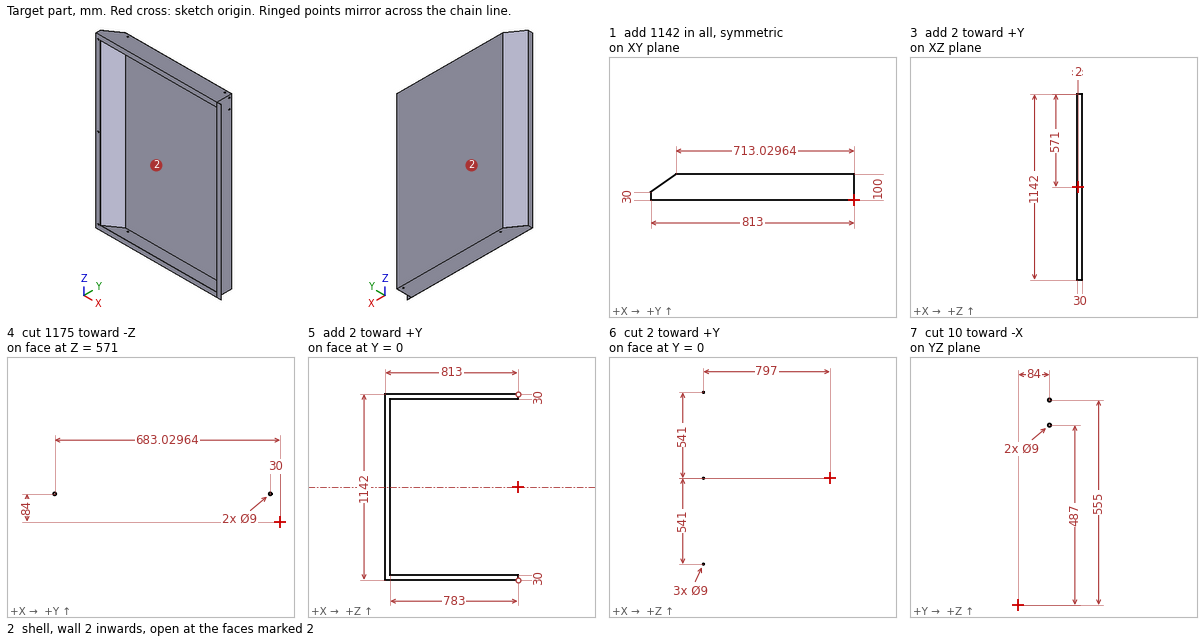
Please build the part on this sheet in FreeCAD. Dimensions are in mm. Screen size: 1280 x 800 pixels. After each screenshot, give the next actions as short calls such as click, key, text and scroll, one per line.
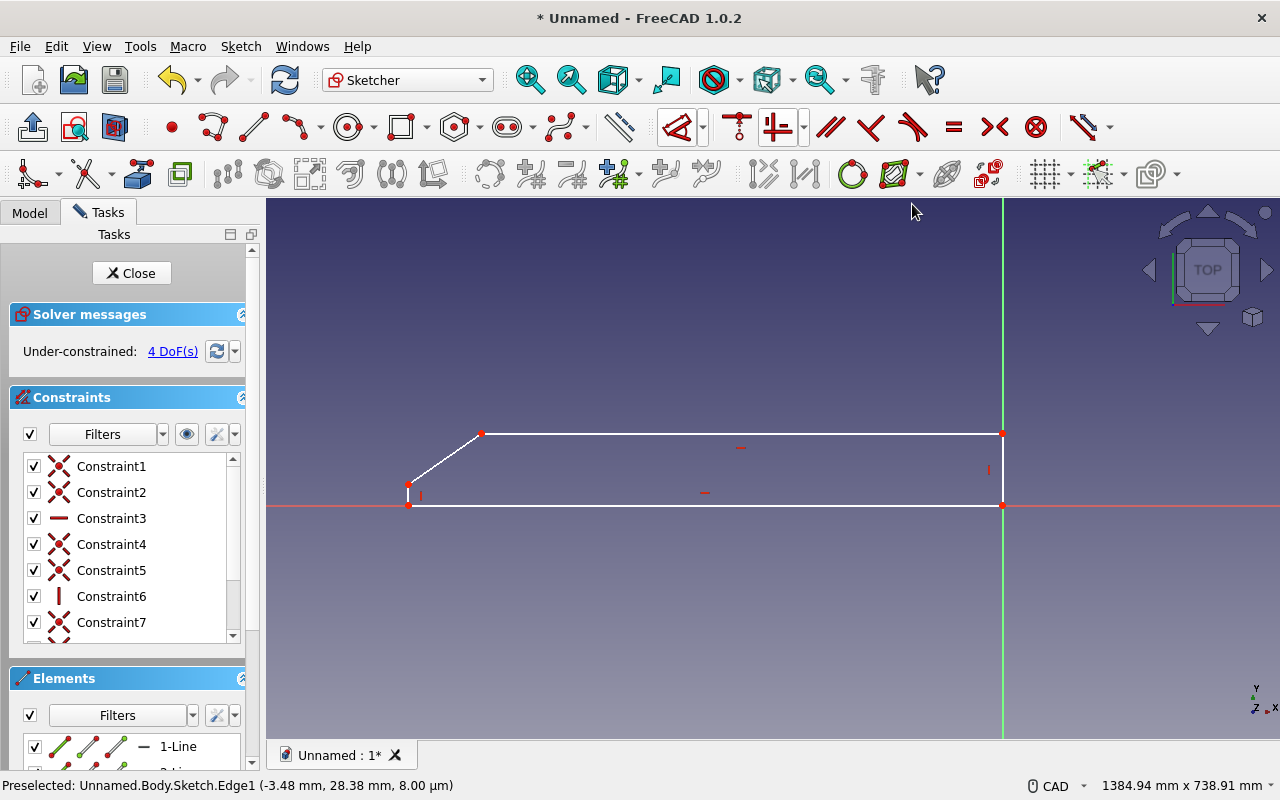
scroll(408, 495, up, 3)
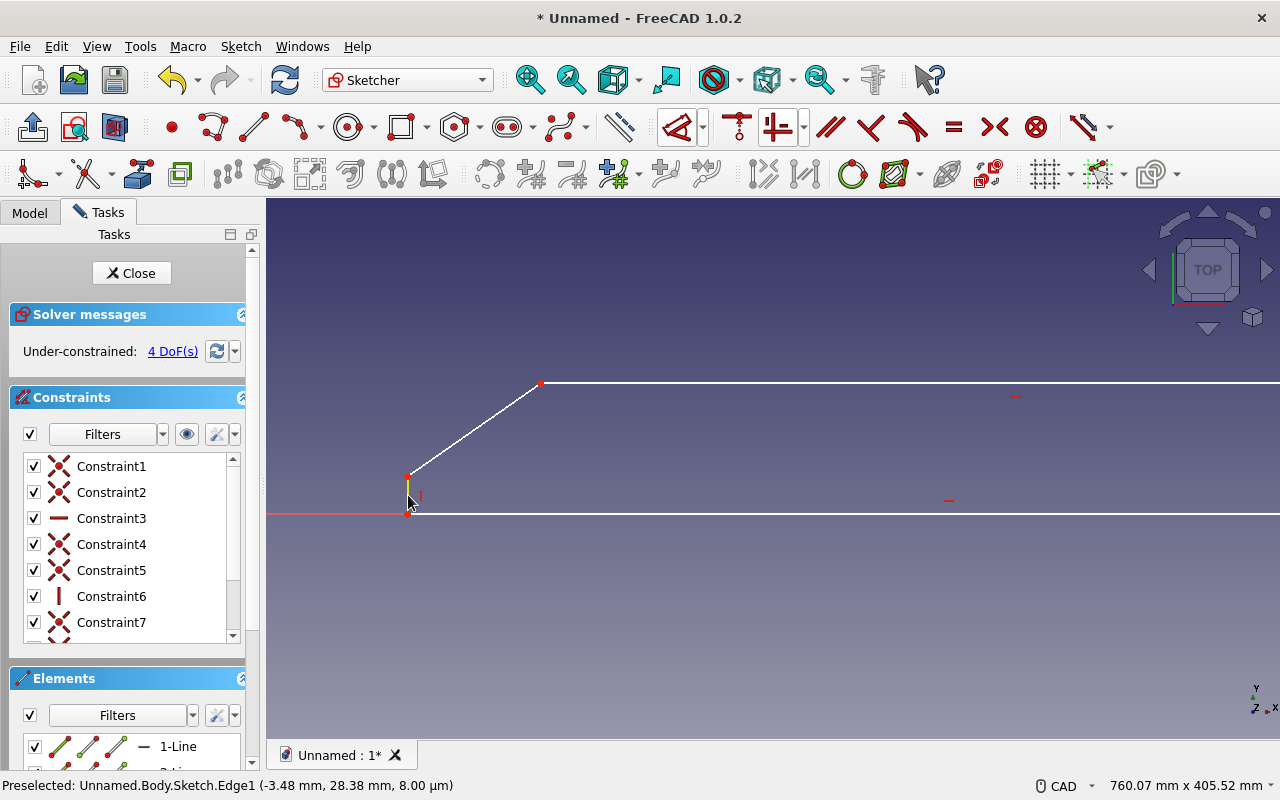
click(408, 495)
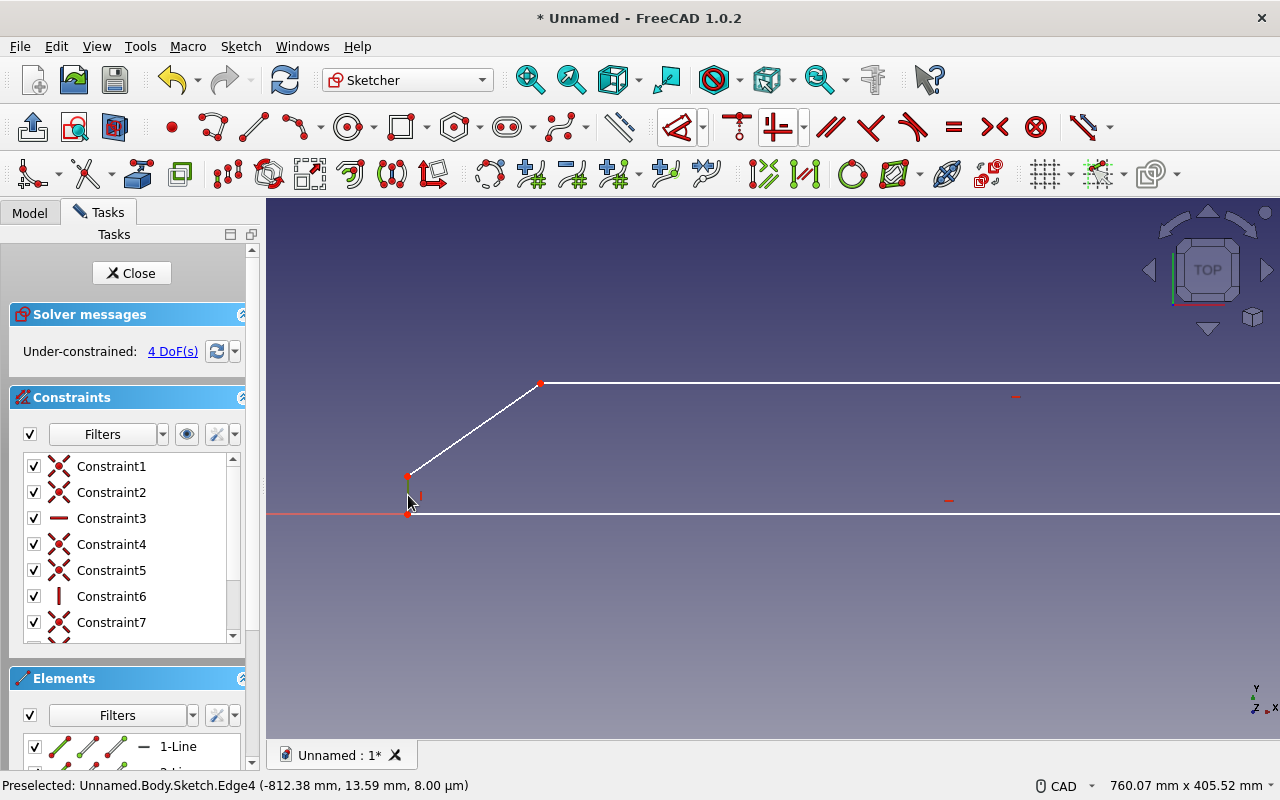
key(i)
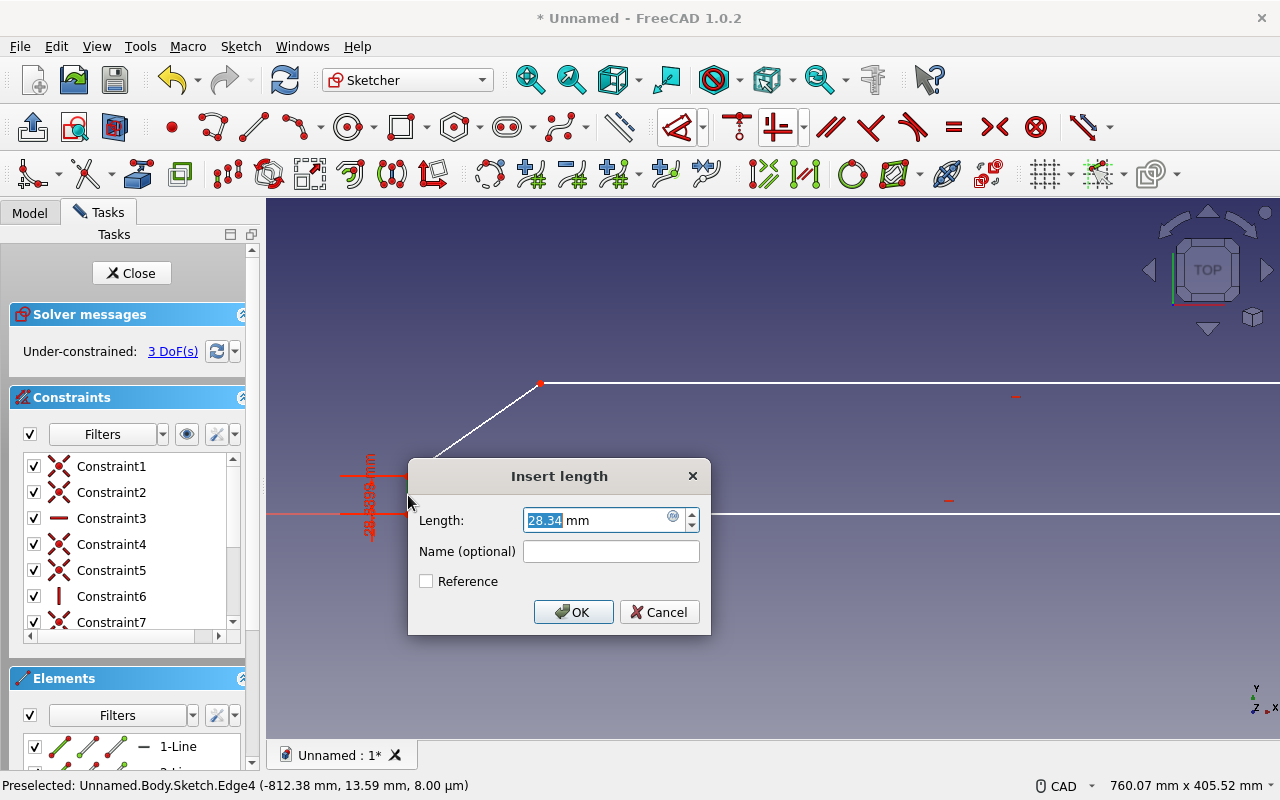
text(30)
key(Return)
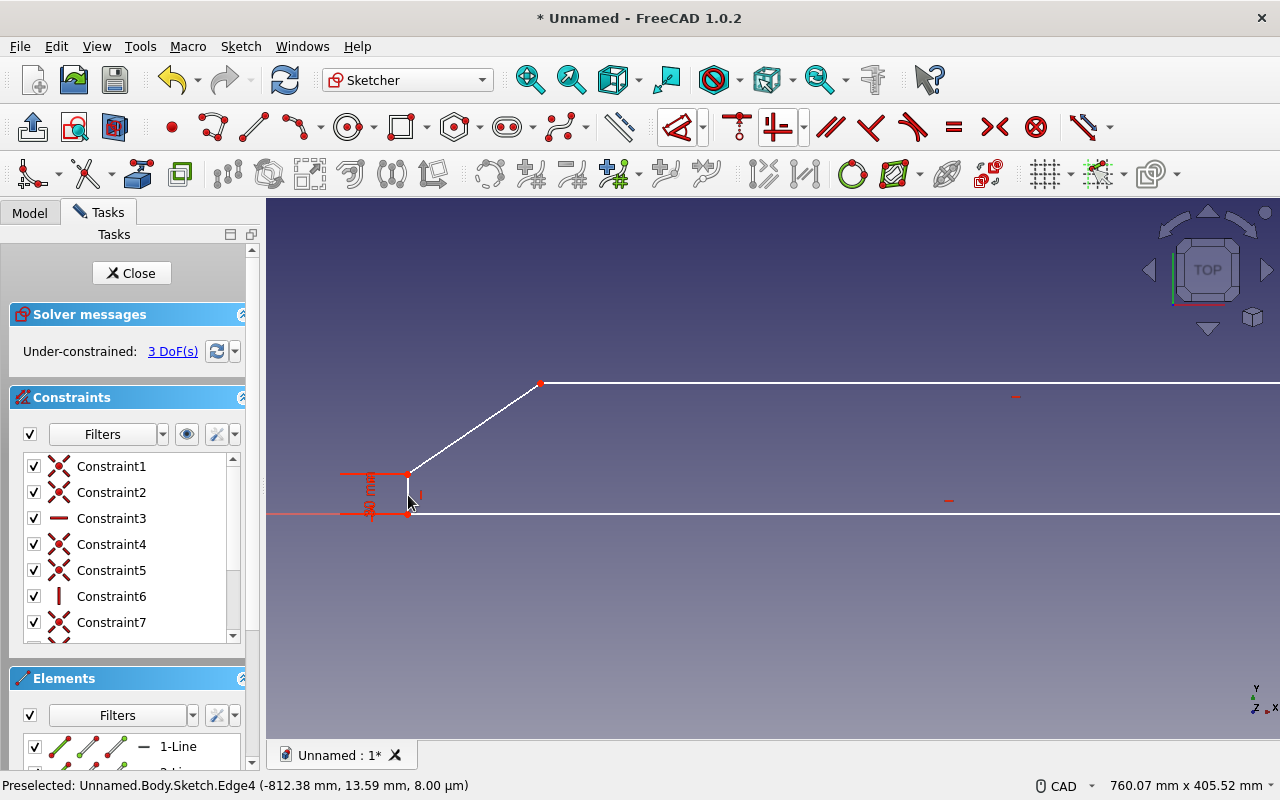
scroll(407, 494, down, 3)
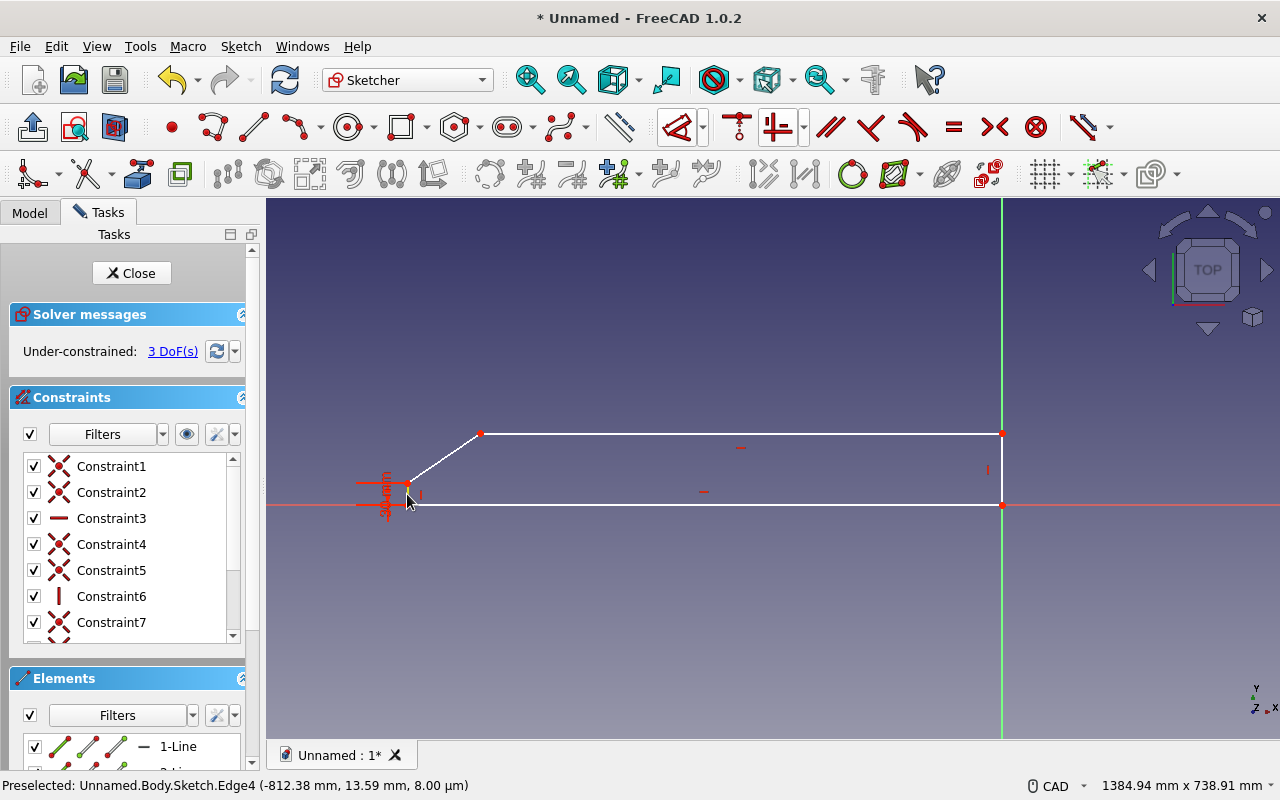
click(1002, 484)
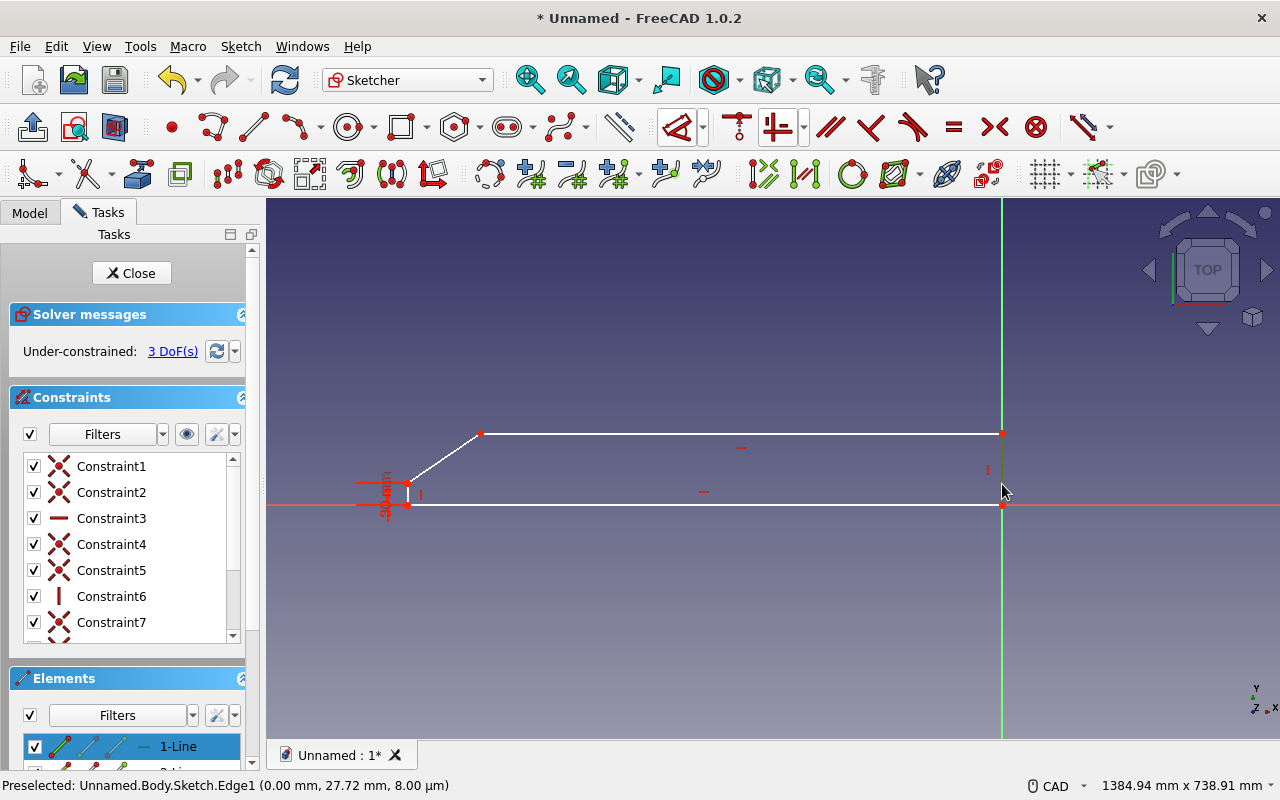
key(i)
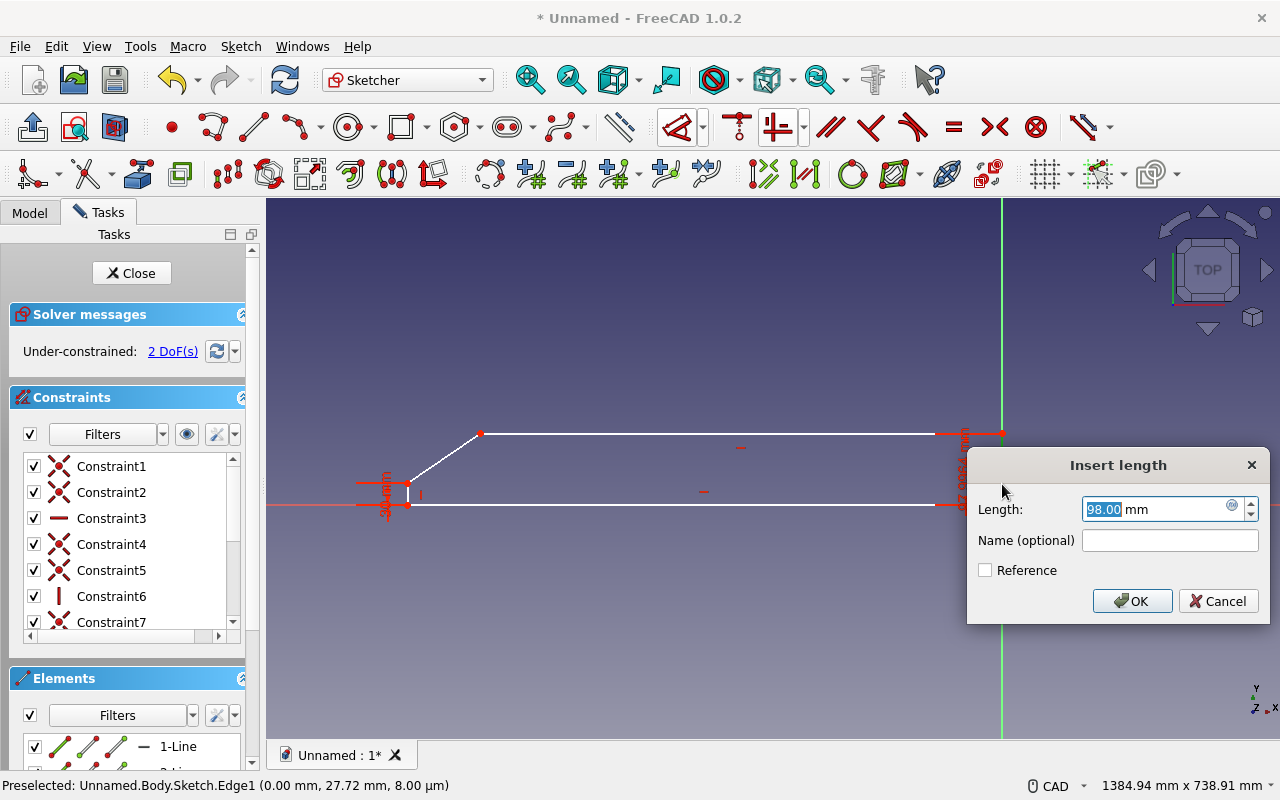
text(100)
key(Return)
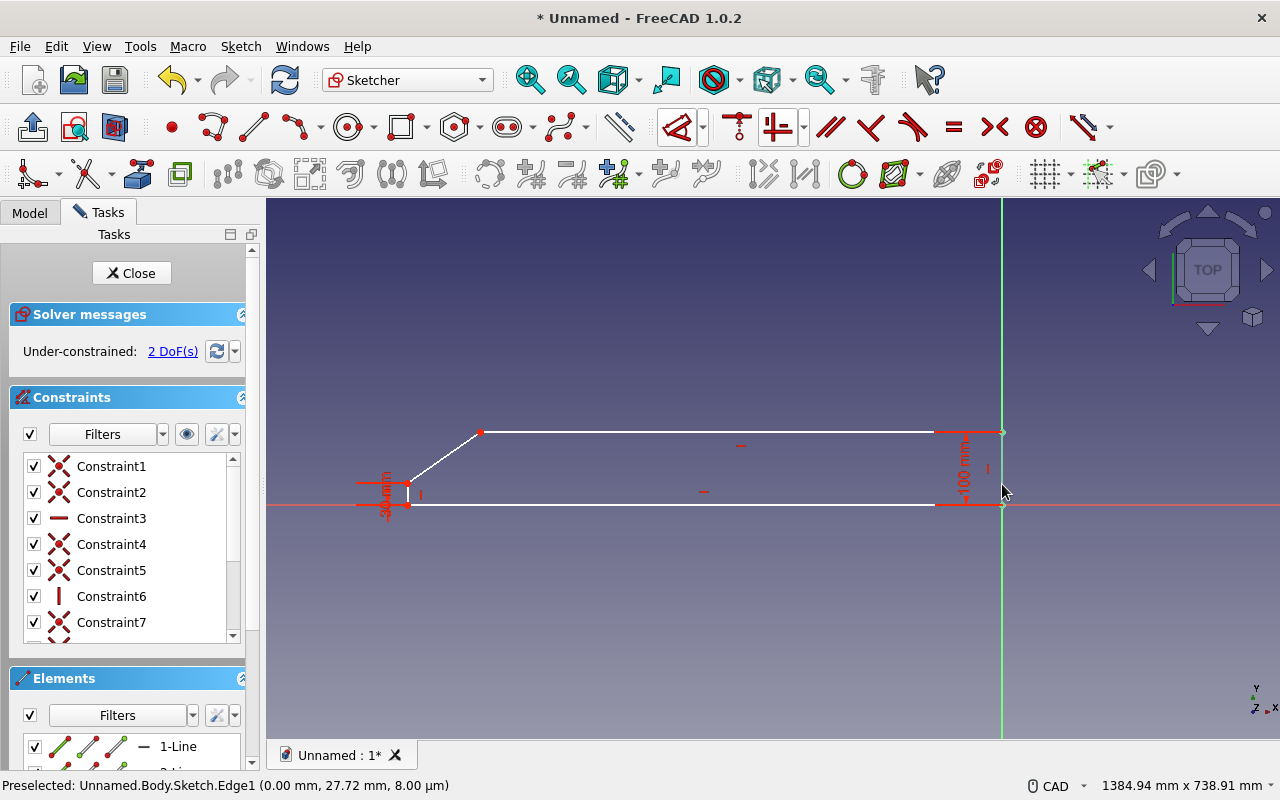
click(586, 505)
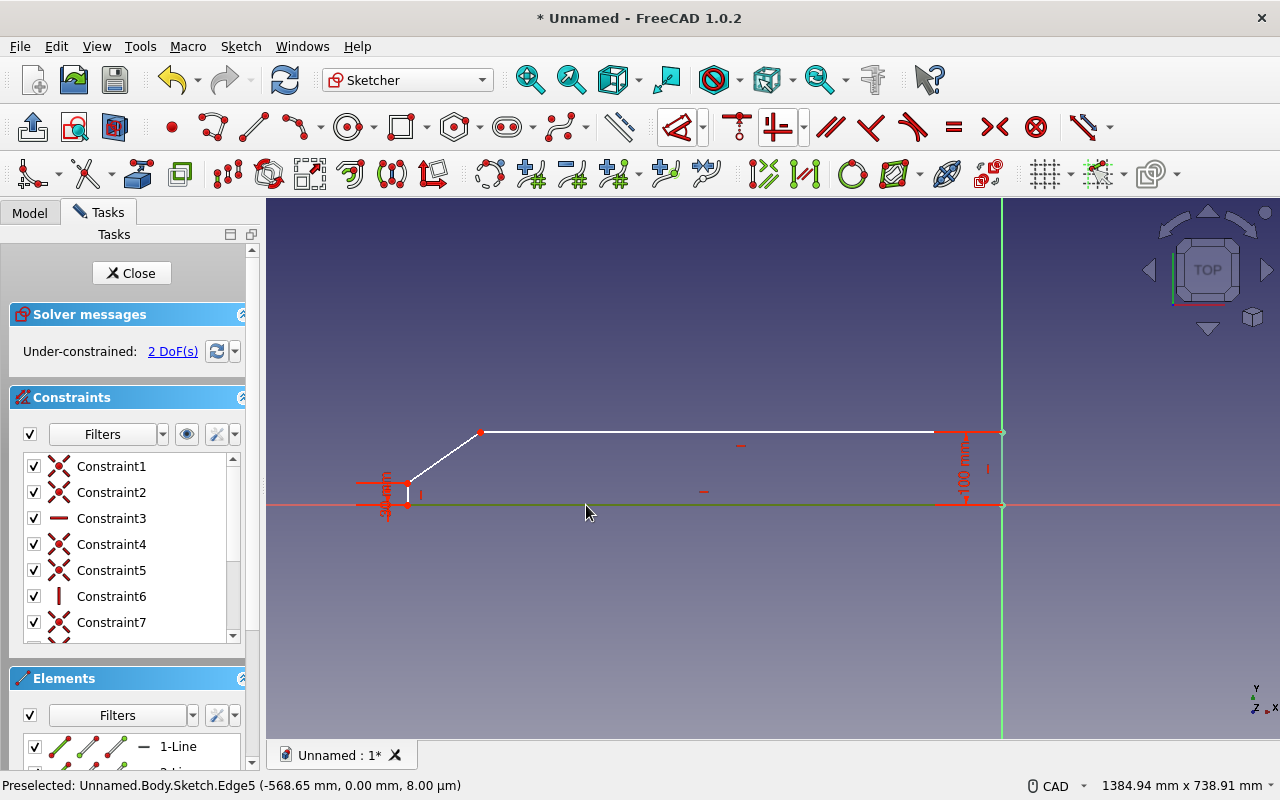
click(702, 128)